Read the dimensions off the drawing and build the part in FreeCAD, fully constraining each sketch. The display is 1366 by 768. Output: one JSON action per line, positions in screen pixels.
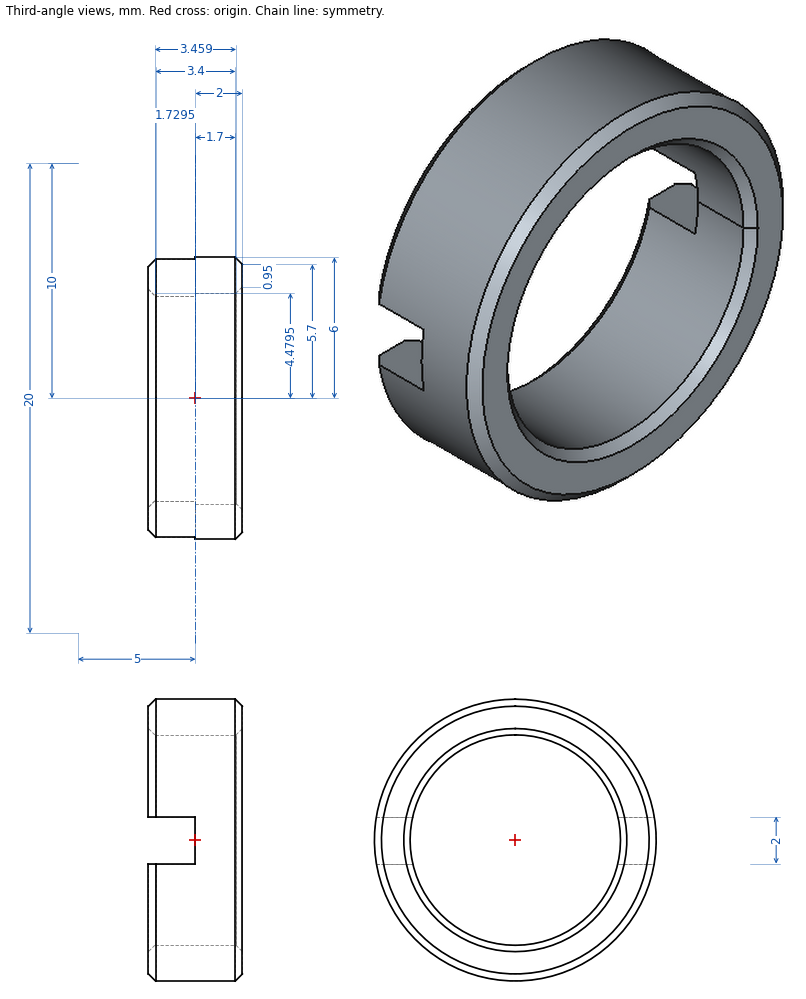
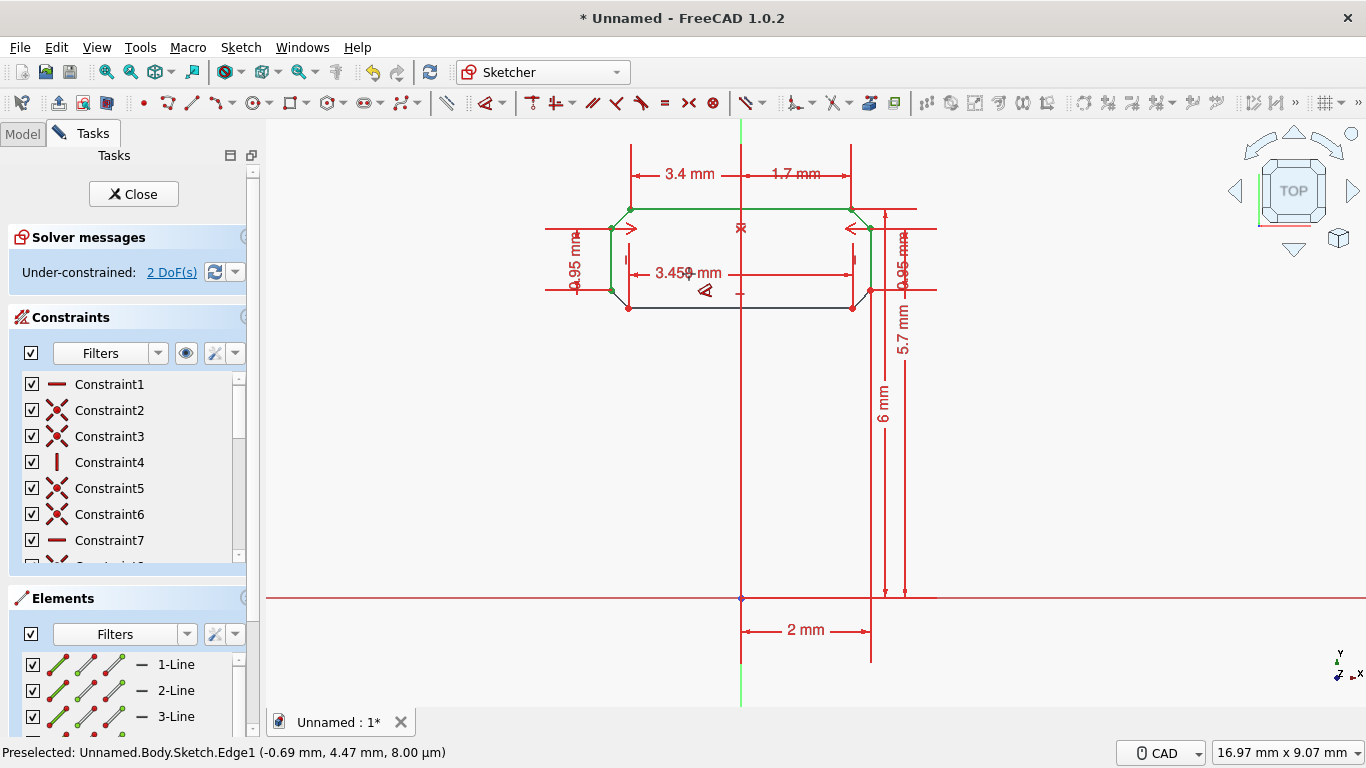
{"action": "left_click", "coordinate": [629, 308]}
{"action": "left_click", "coordinate": [685, 632]}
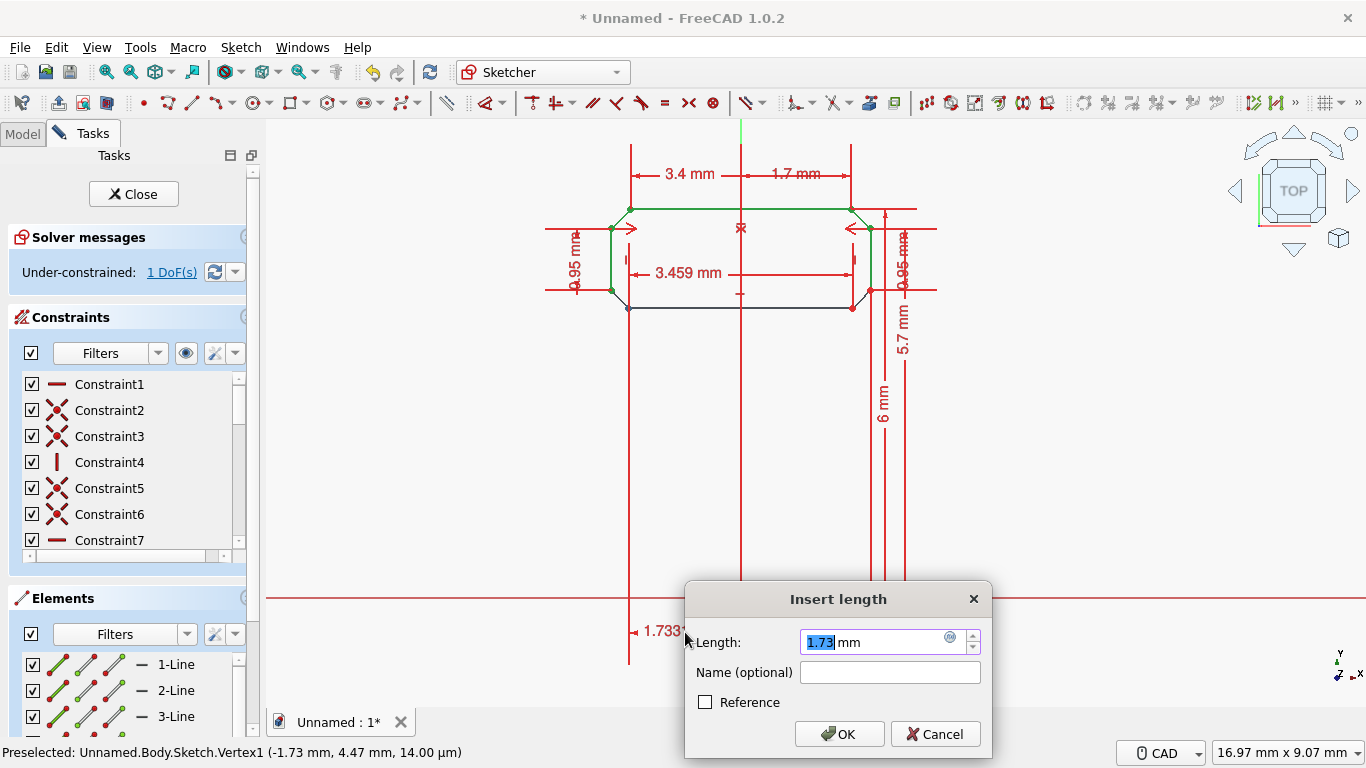
{"action": "type", "text": "1.7295"}
{"action": "key", "text": "Return"}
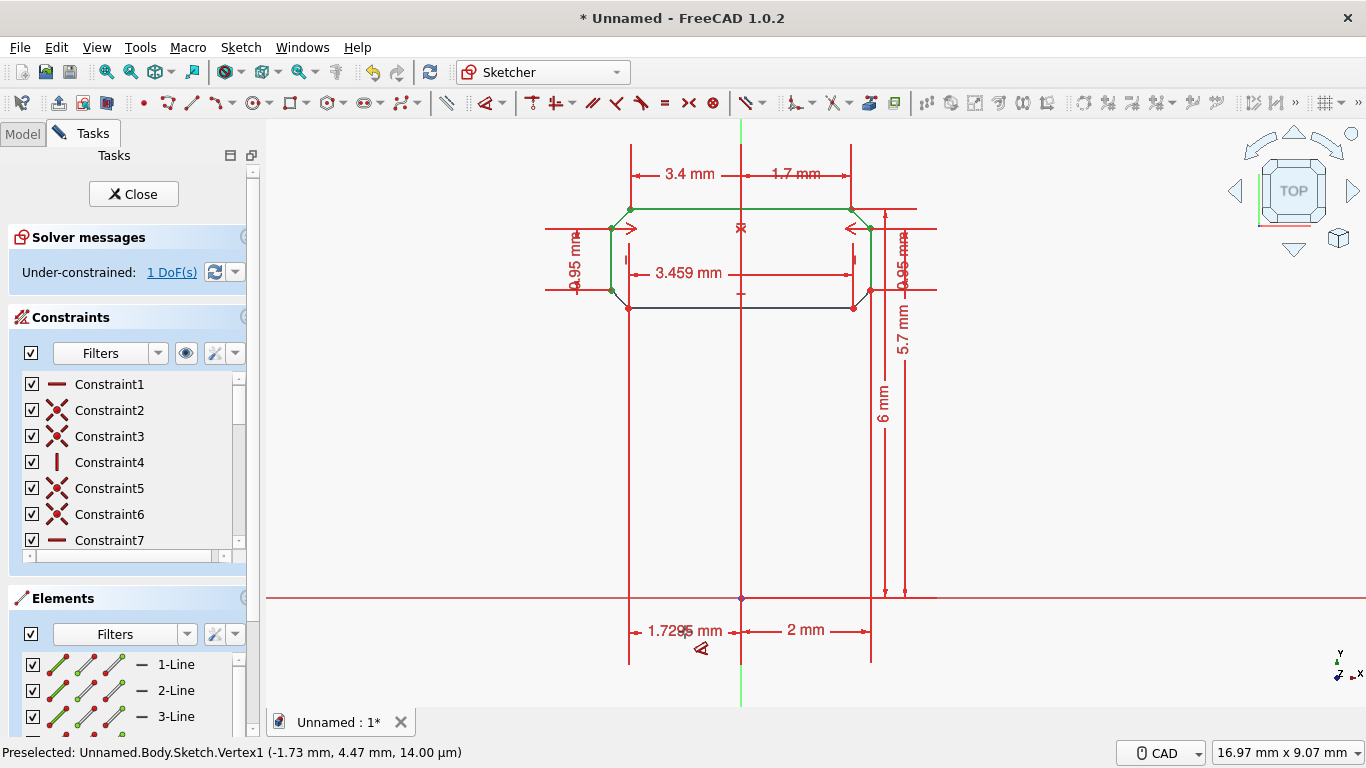
{"action": "left_click", "coordinate": [629, 308]}
{"action": "left_click", "coordinate": [595, 453]}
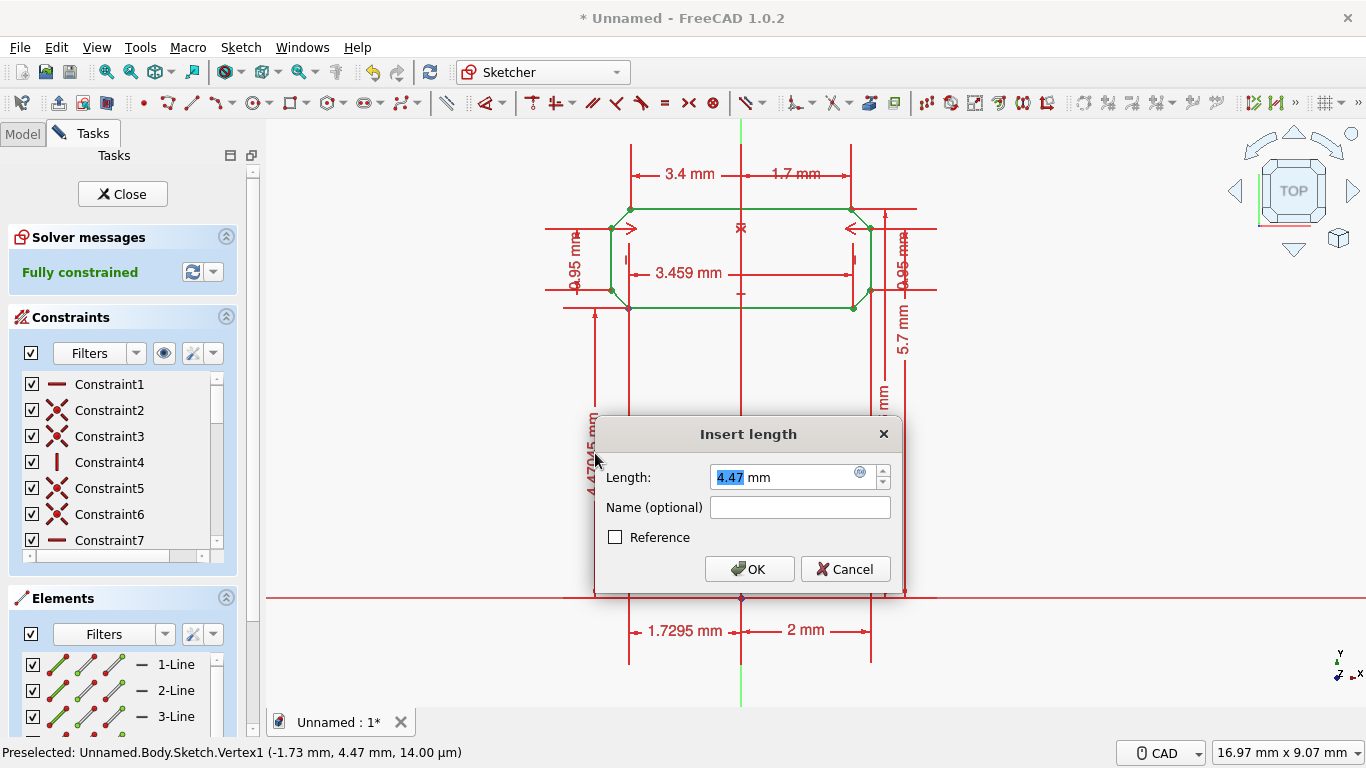
{"action": "type", "text": "4.4795"}
{"action": "key", "text": "Return"}
{"action": "key", "text": "Escape"}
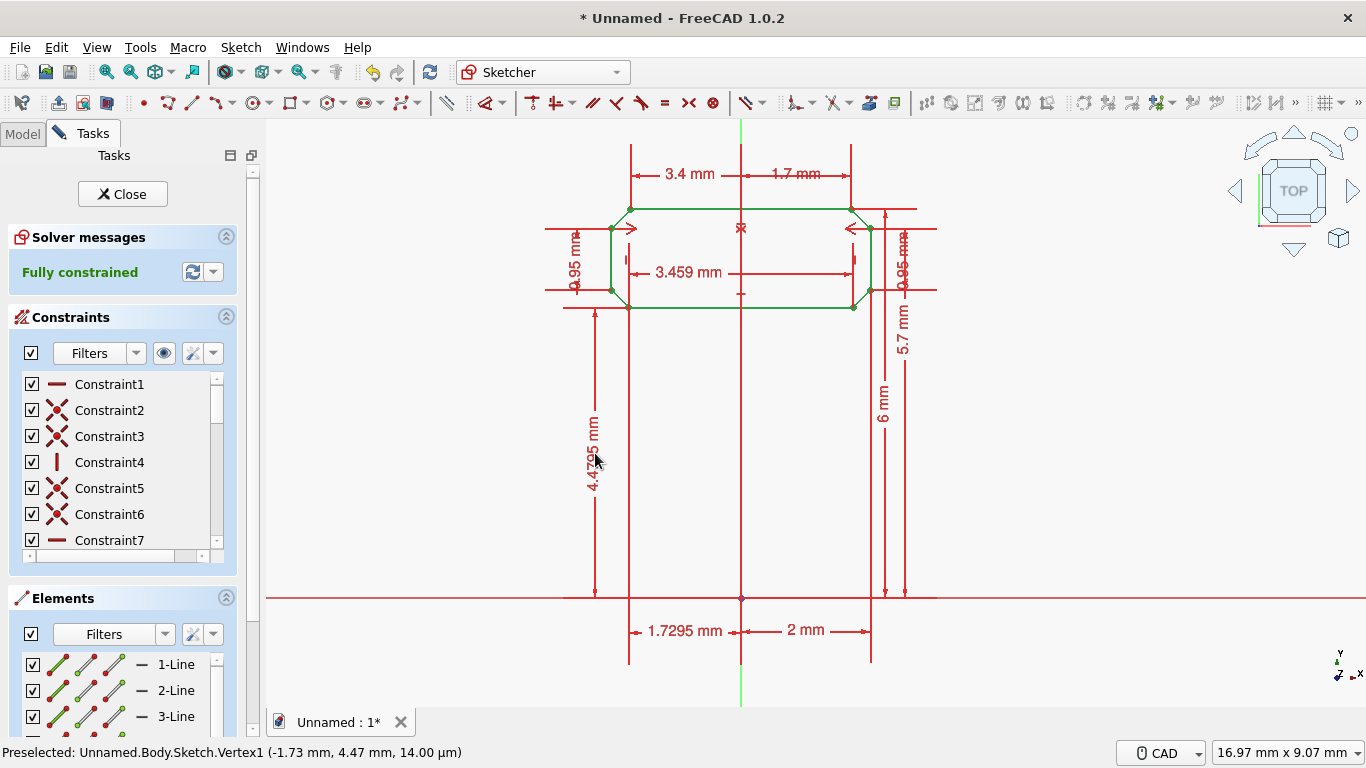
{"action": "left_click", "coordinate": [123, 194]}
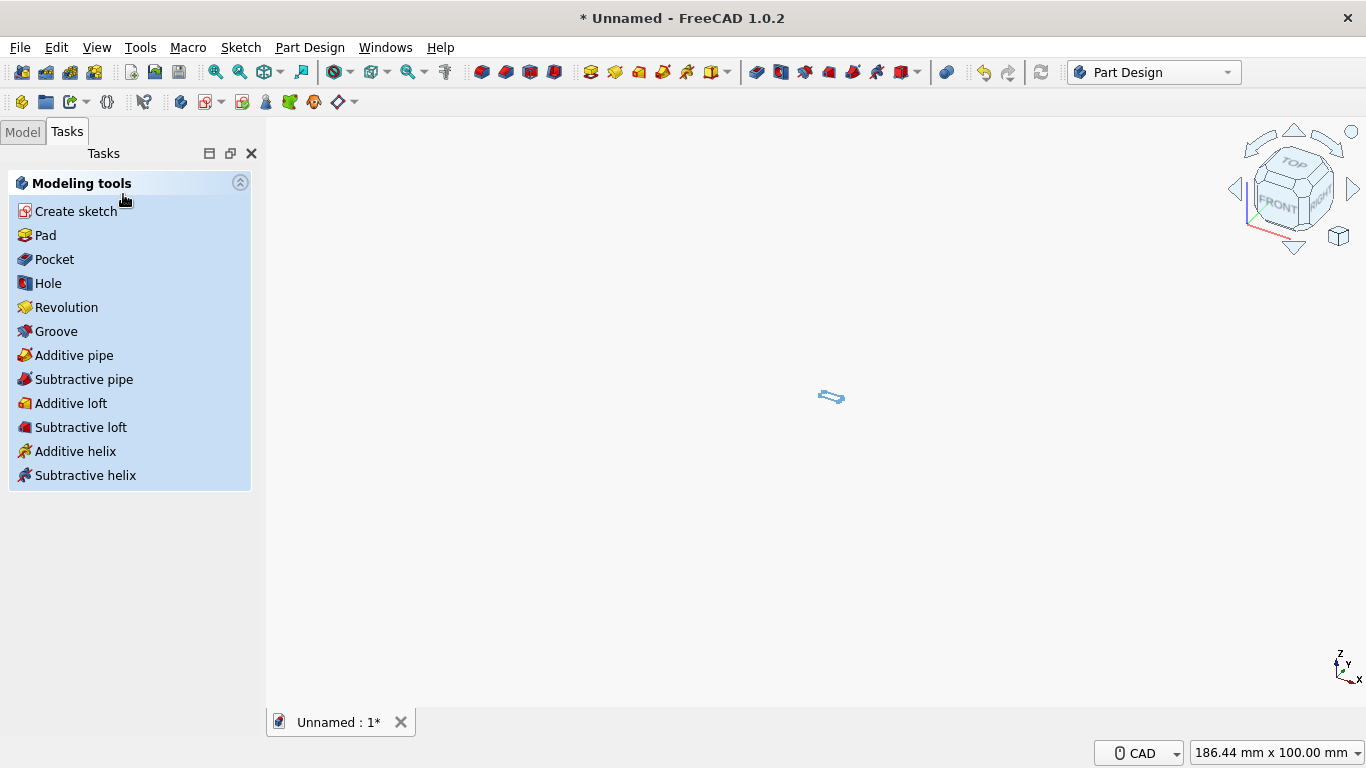
{"action": "left_click", "coordinate": [616, 72]}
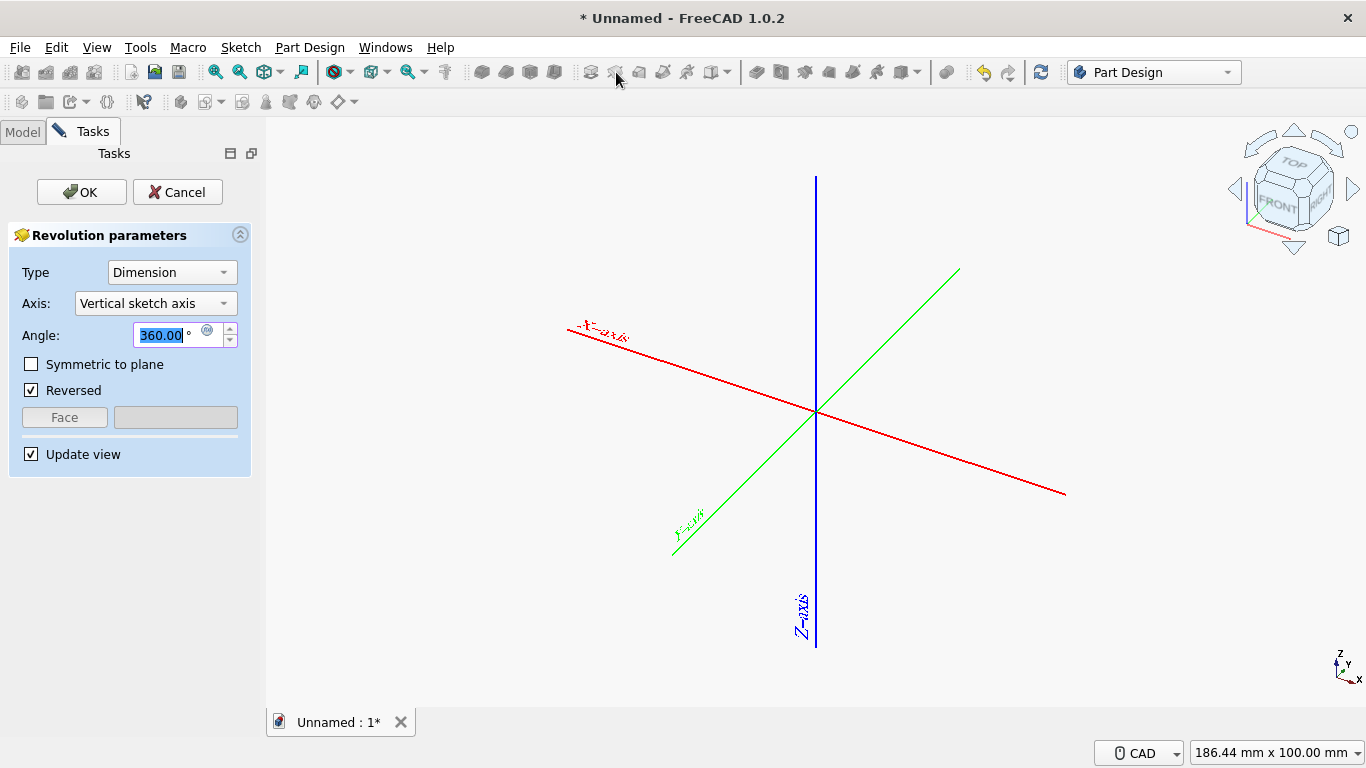
{"action": "left_click", "coordinate": [156, 304]}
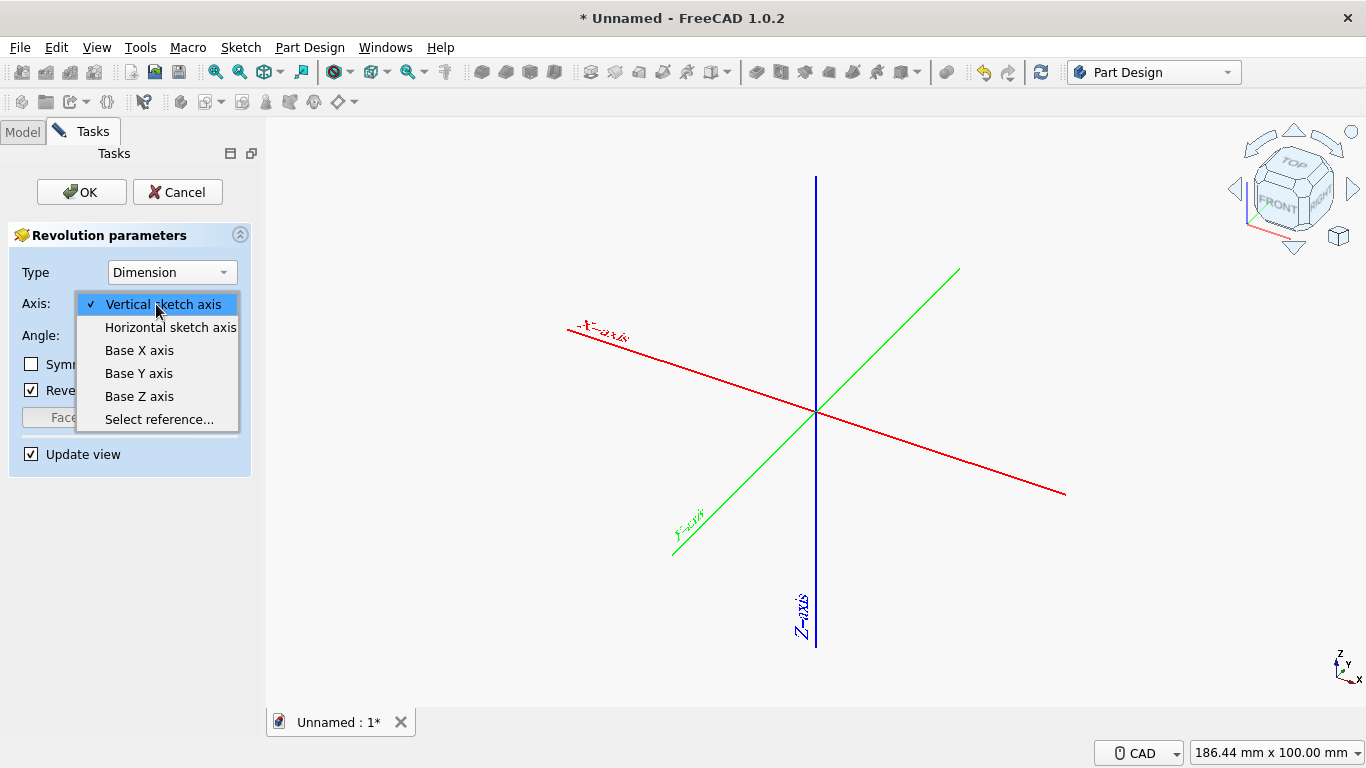
{"action": "left_click", "coordinate": [156, 328]}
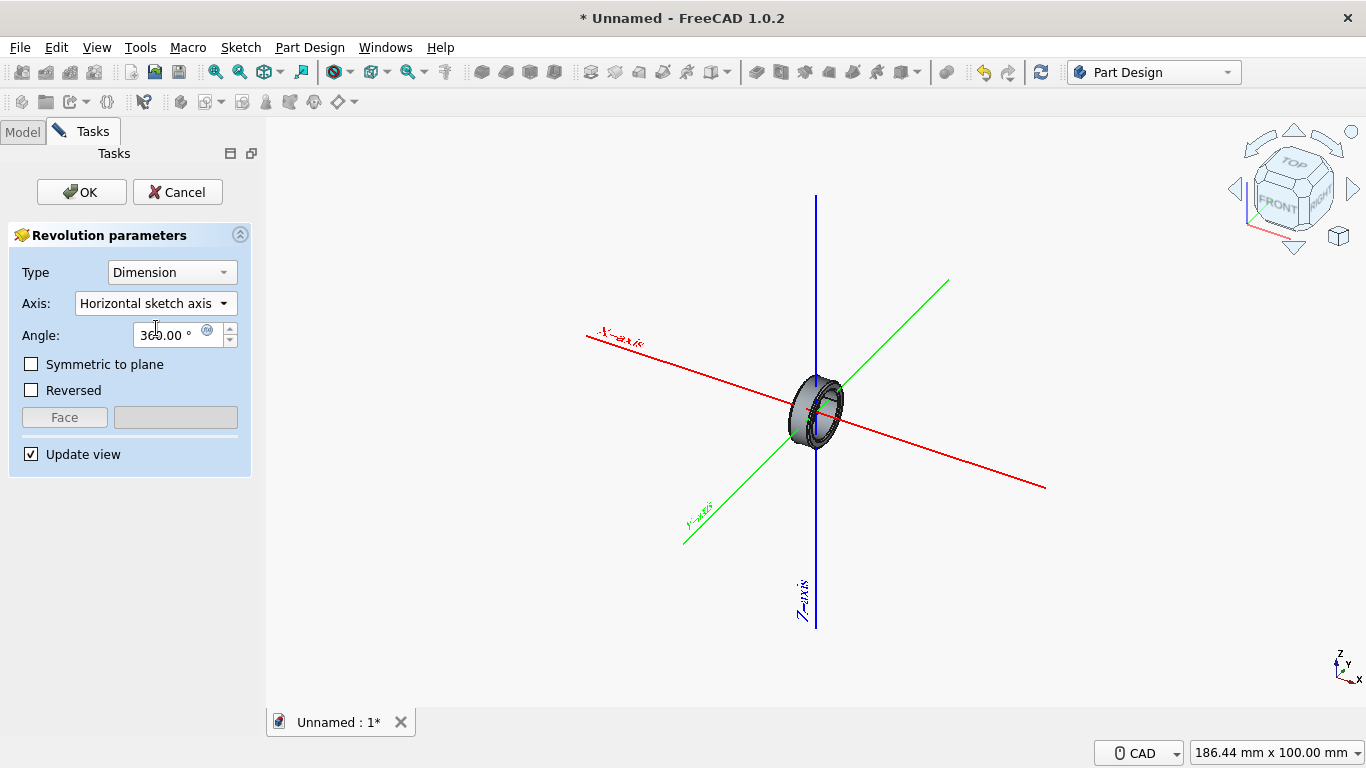
{"action": "left_click", "coordinate": [82, 192]}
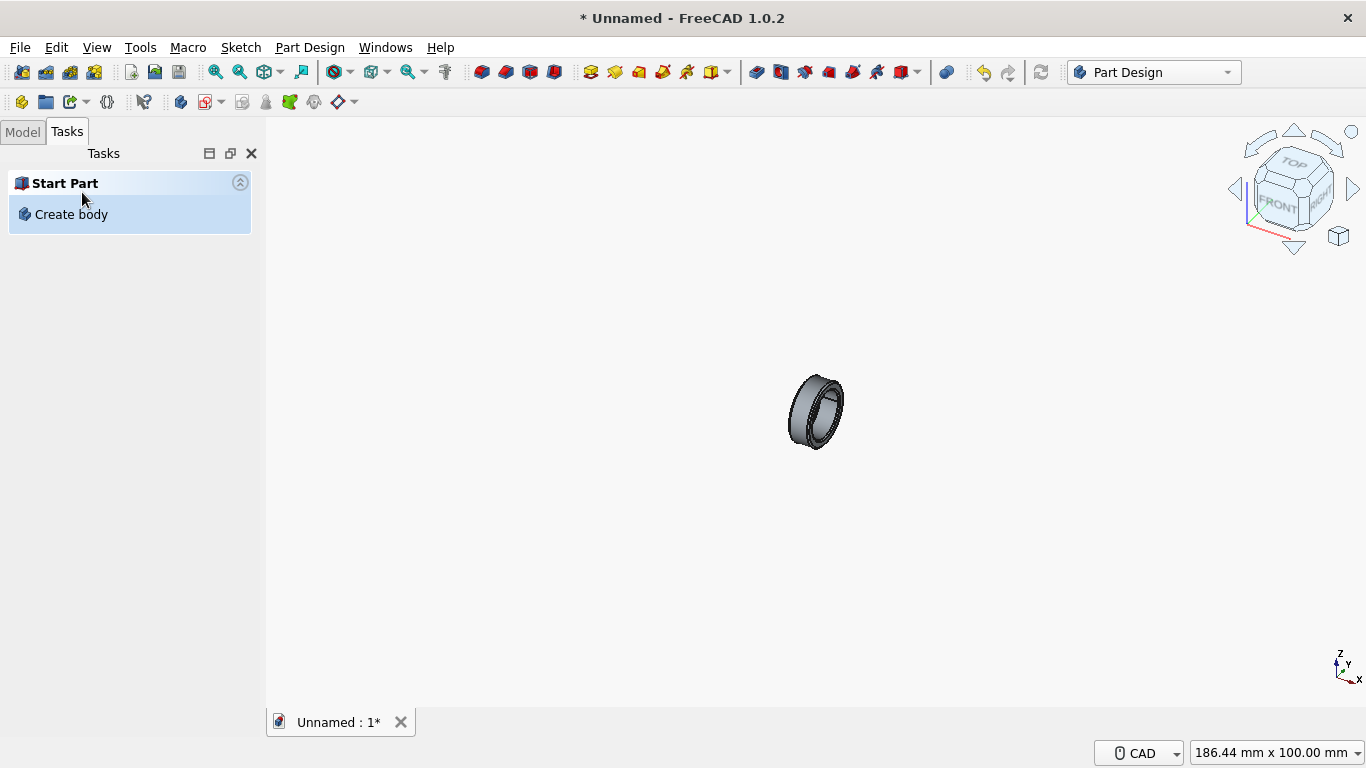
{"action": "left_click", "coordinate": [216, 72]}